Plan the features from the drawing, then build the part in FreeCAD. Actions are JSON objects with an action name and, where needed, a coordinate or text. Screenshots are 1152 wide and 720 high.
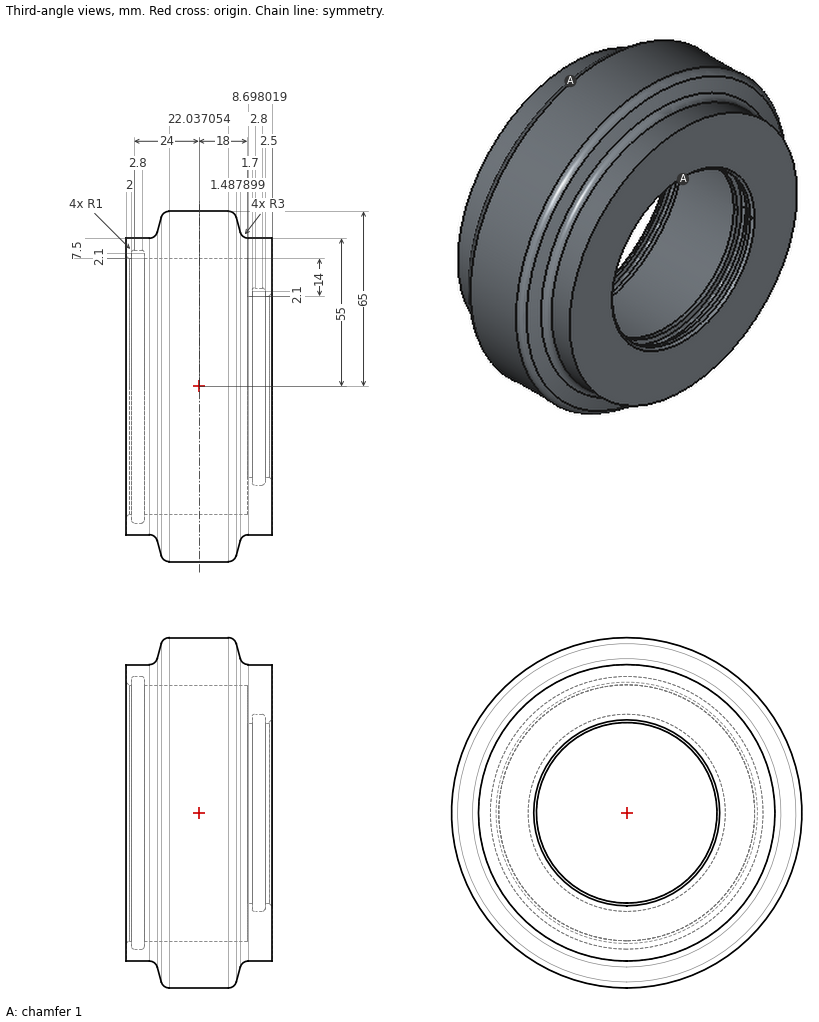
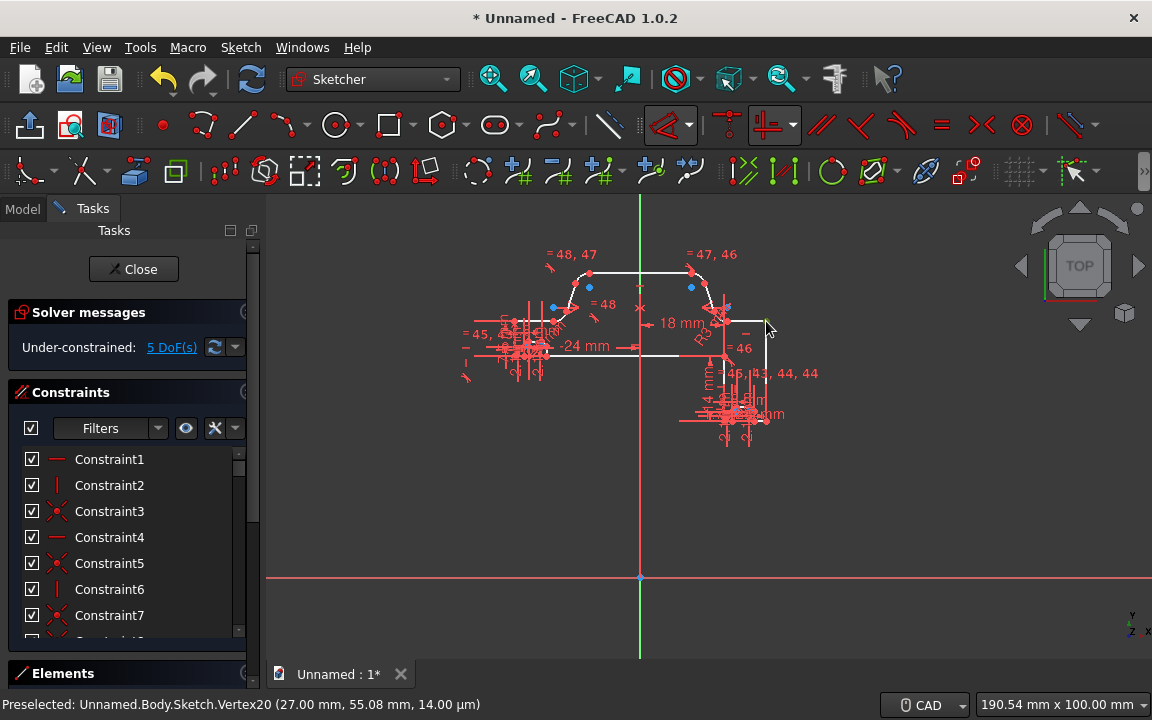
{"action": "key", "text": "i"}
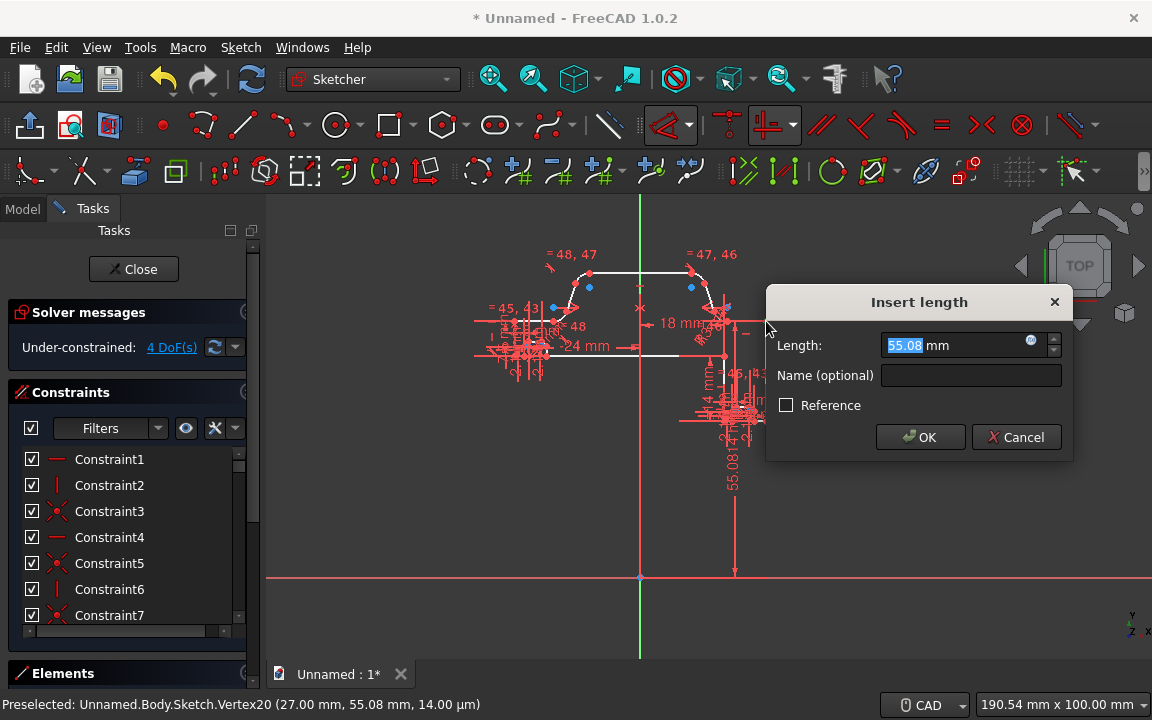
{"action": "type", "text": "55"}
{"action": "key", "text": "Return"}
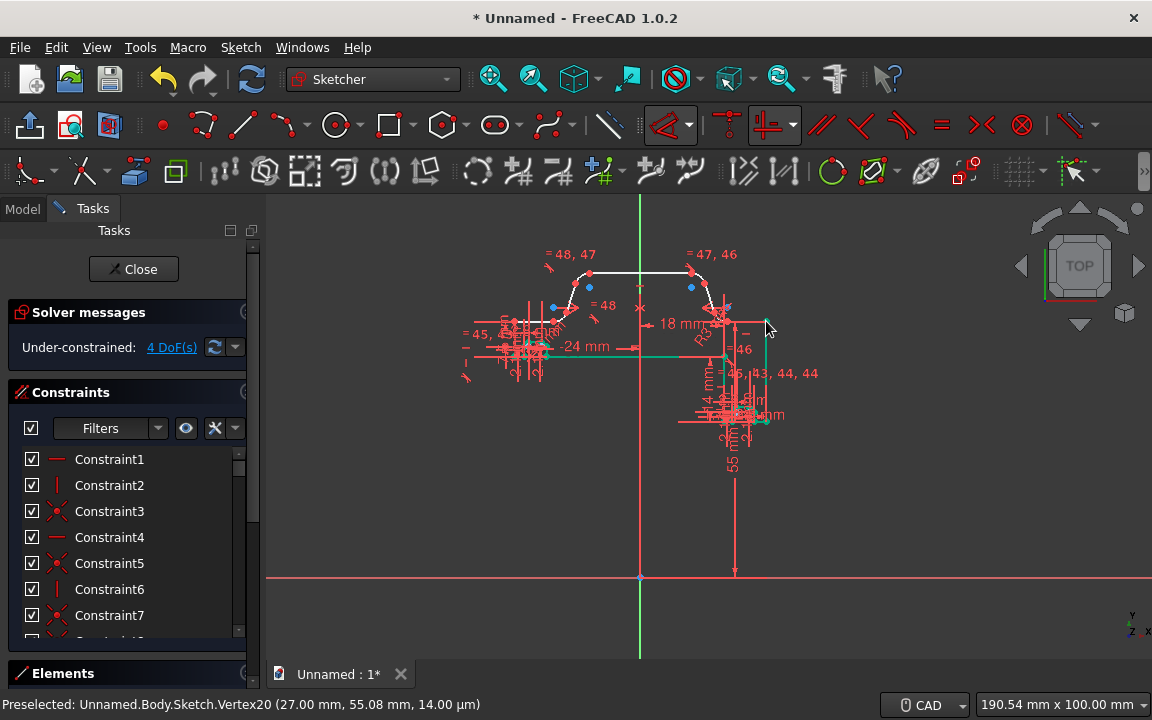
{"action": "left_click", "coordinate": [692, 273]}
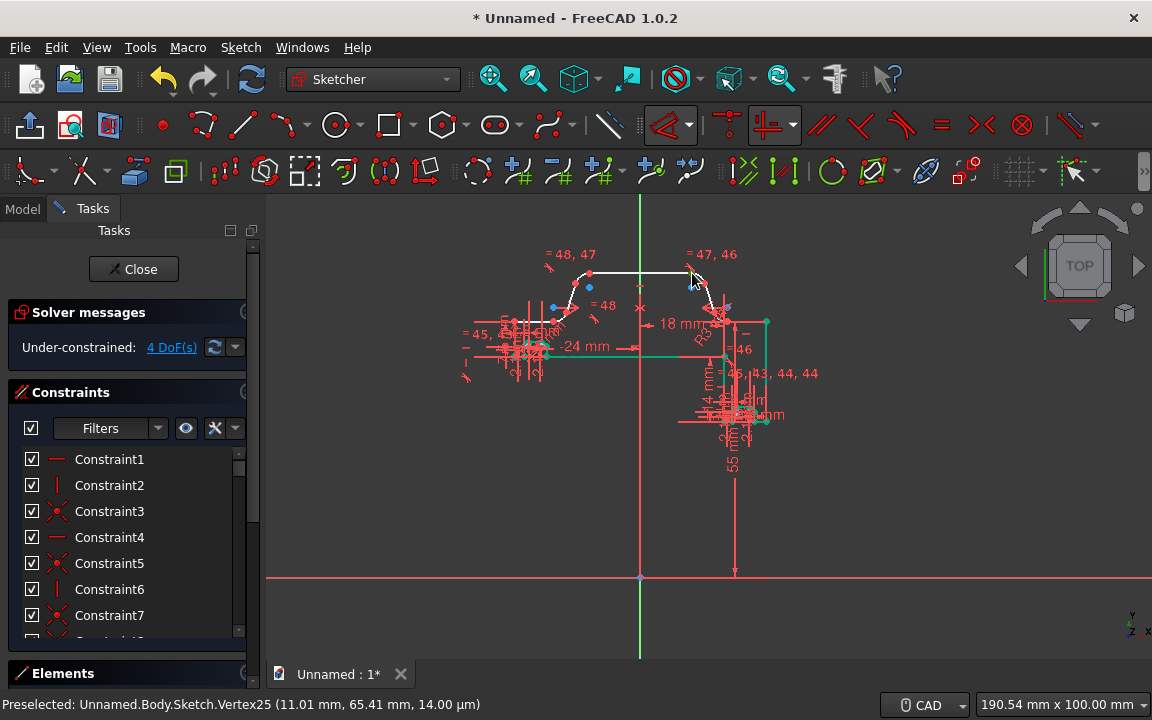
{"action": "key", "text": "i"}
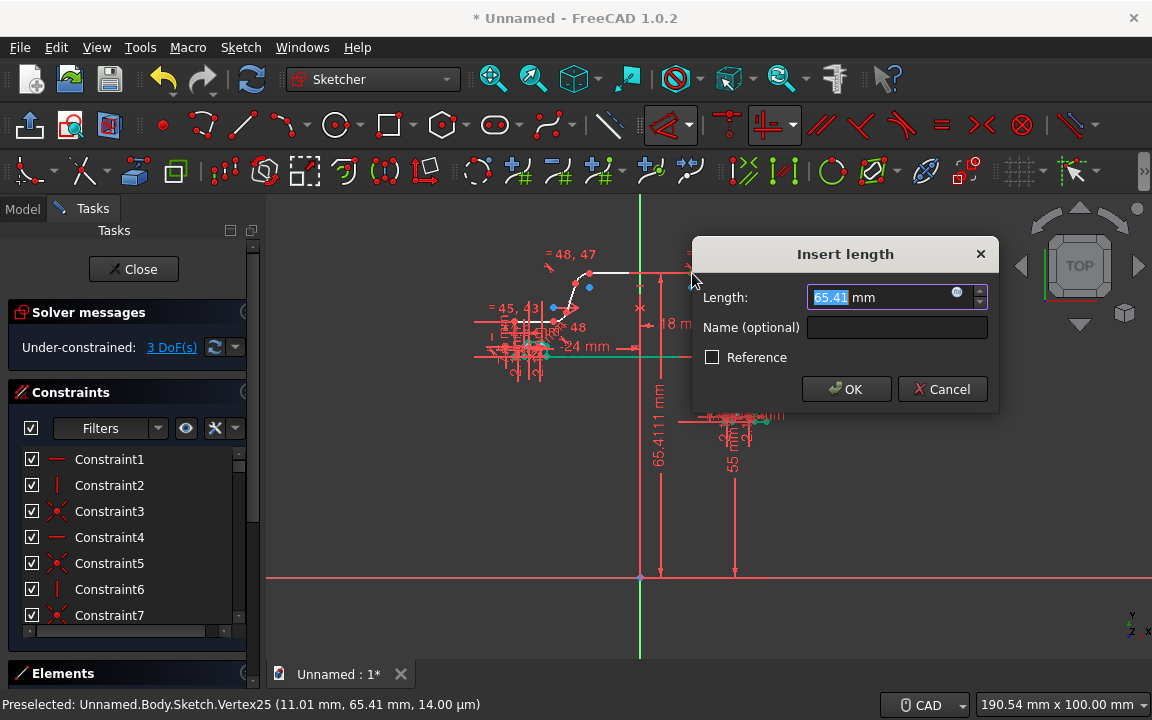
{"action": "type", "text": "65"}
{"action": "key", "text": "Return"}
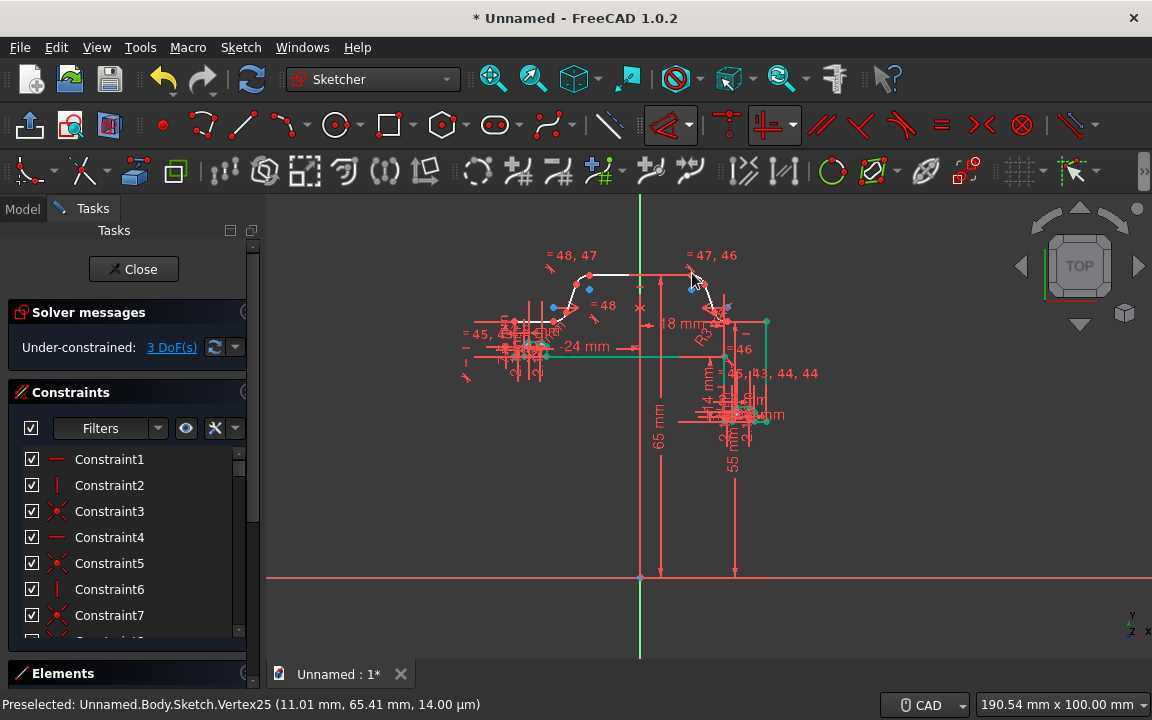
{"action": "left_click", "coordinate": [754, 322]}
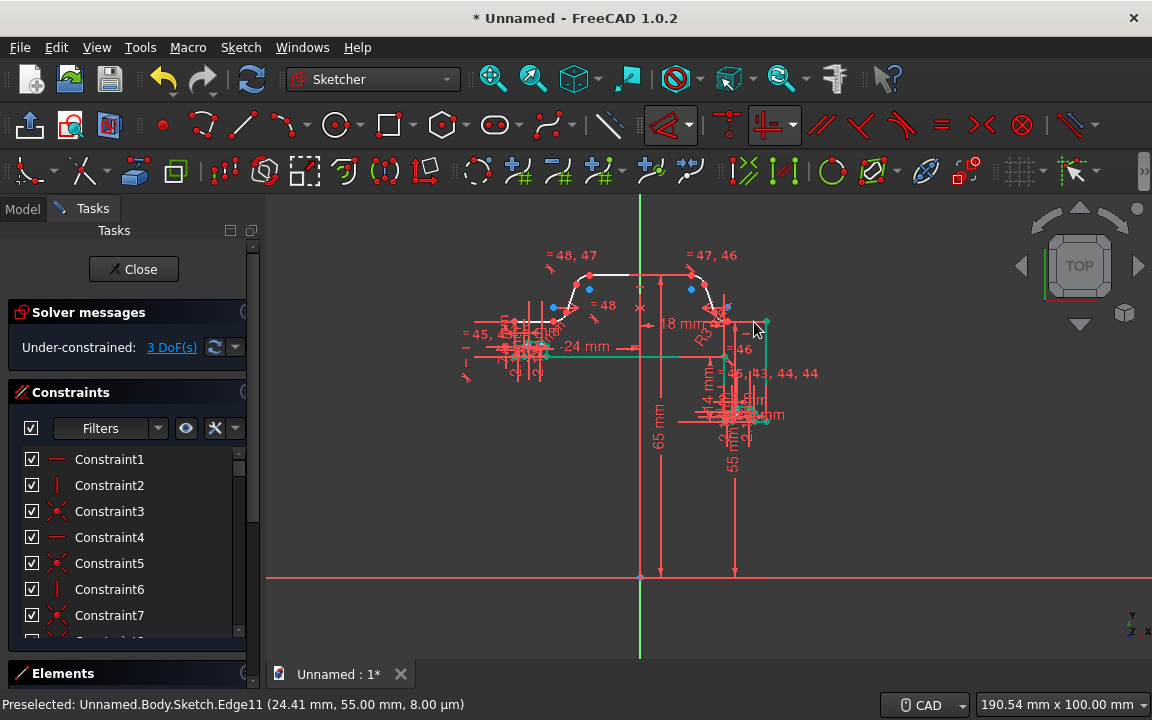
{"action": "left_click", "coordinate": [692, 126]}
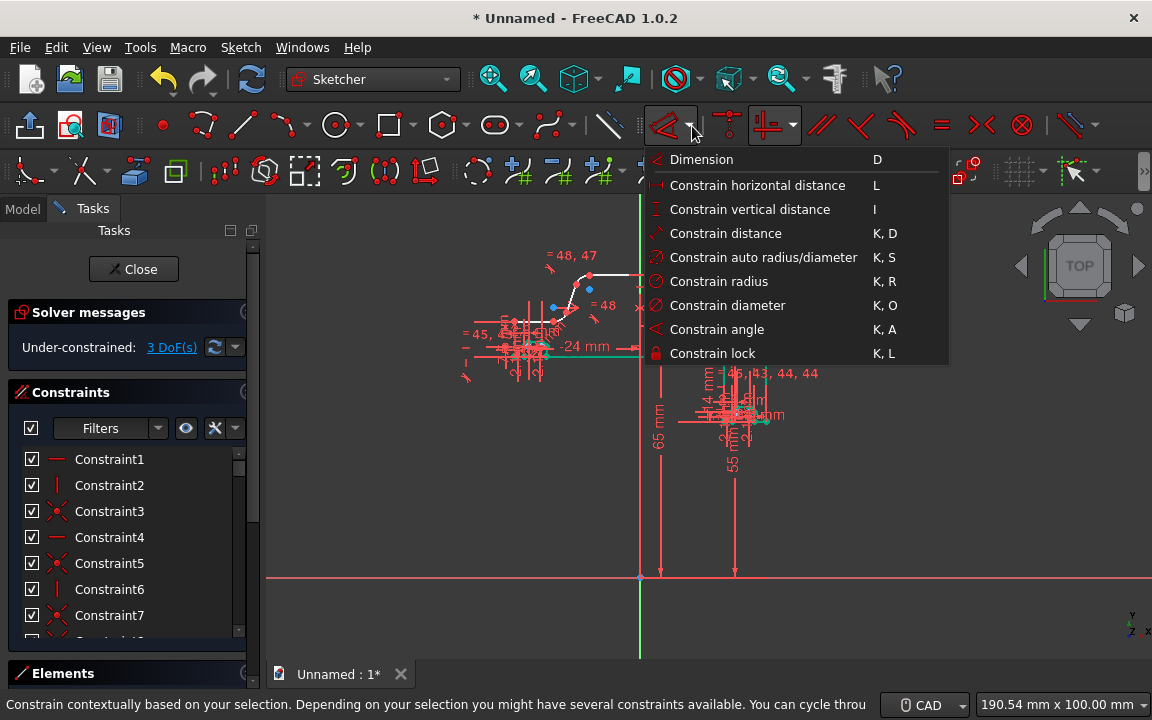
{"action": "left_click", "coordinate": [797, 185]}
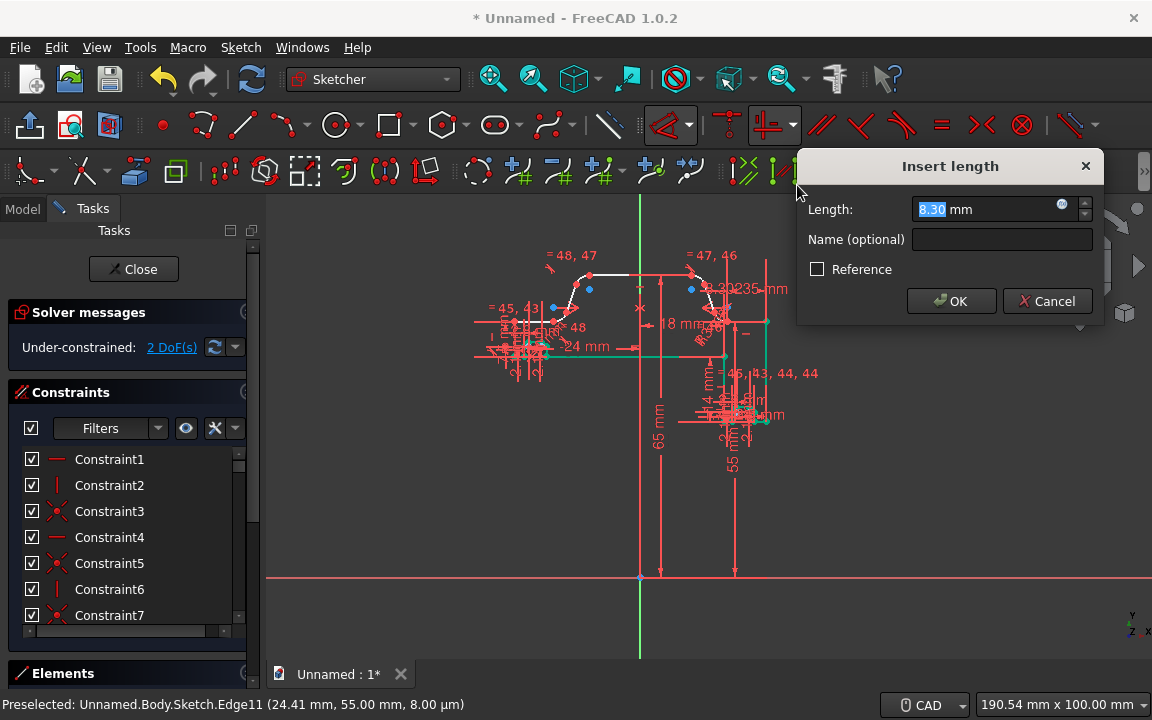
{"action": "type", "text": "8.698019"}
{"action": "key", "text": "Return"}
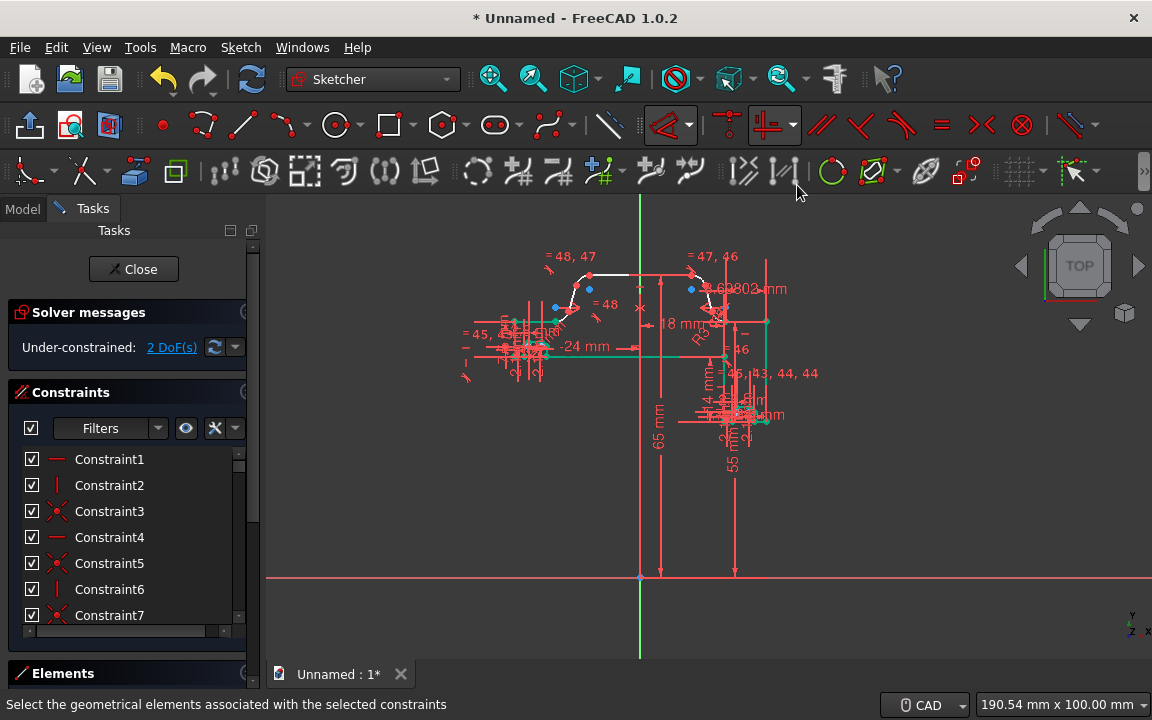
{"action": "left_click", "coordinate": [661, 275]}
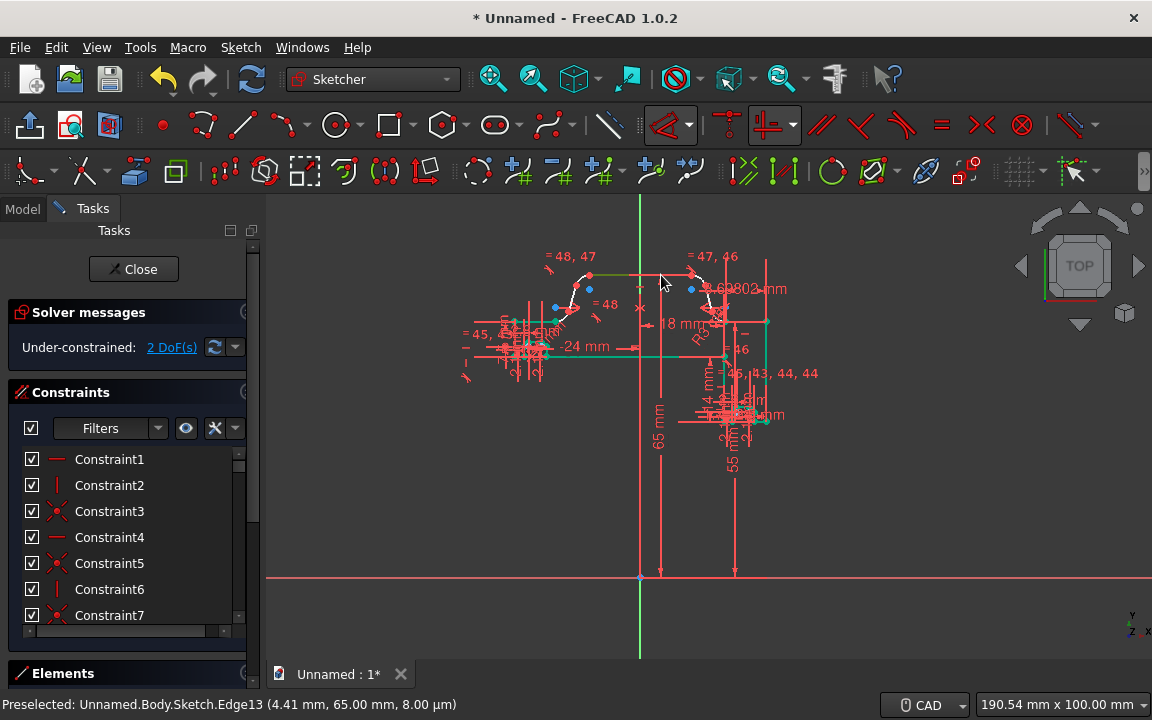
{"action": "key", "text": "l"}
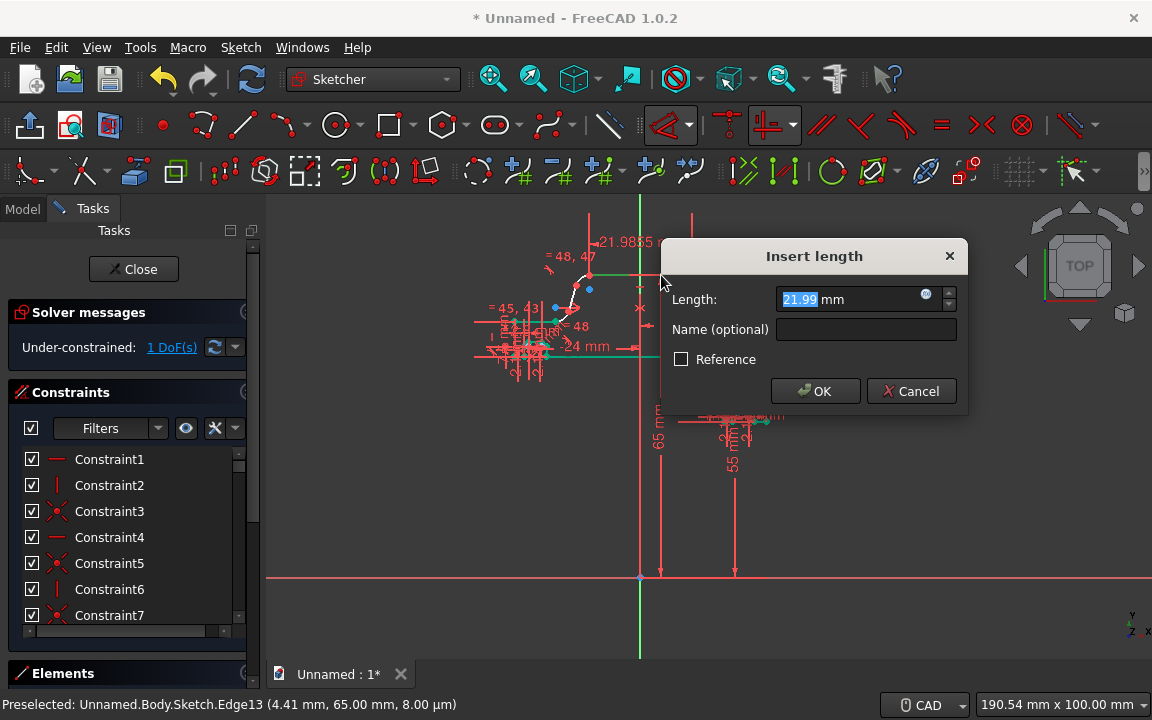
{"action": "type", "text": "22.037054"}
{"action": "key", "text": "Return"}